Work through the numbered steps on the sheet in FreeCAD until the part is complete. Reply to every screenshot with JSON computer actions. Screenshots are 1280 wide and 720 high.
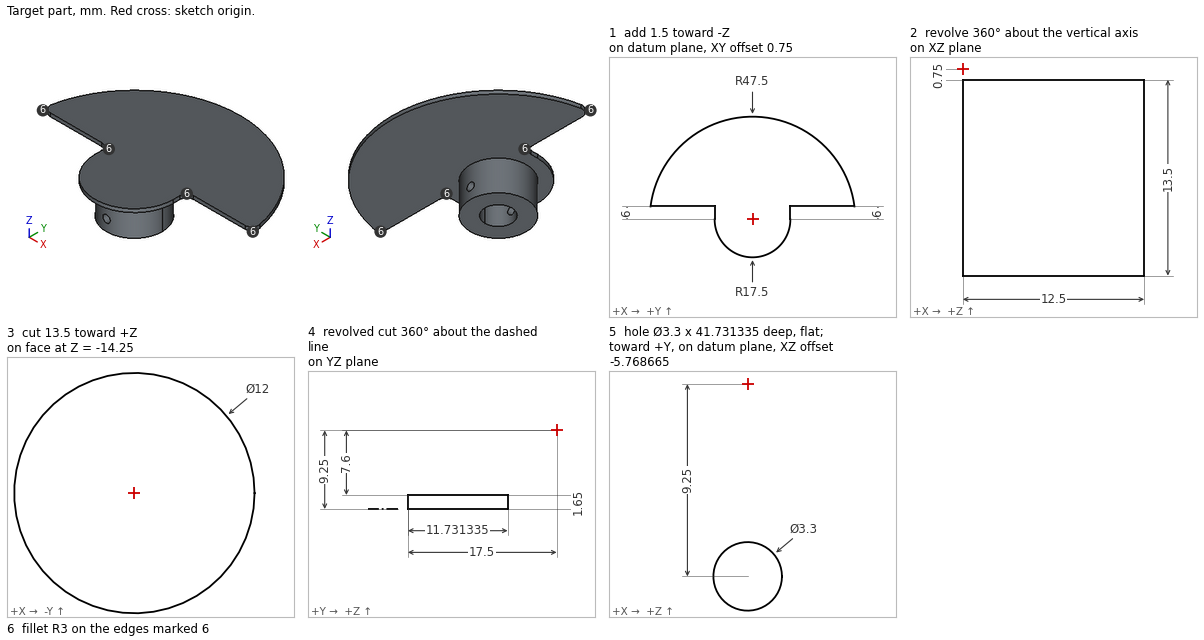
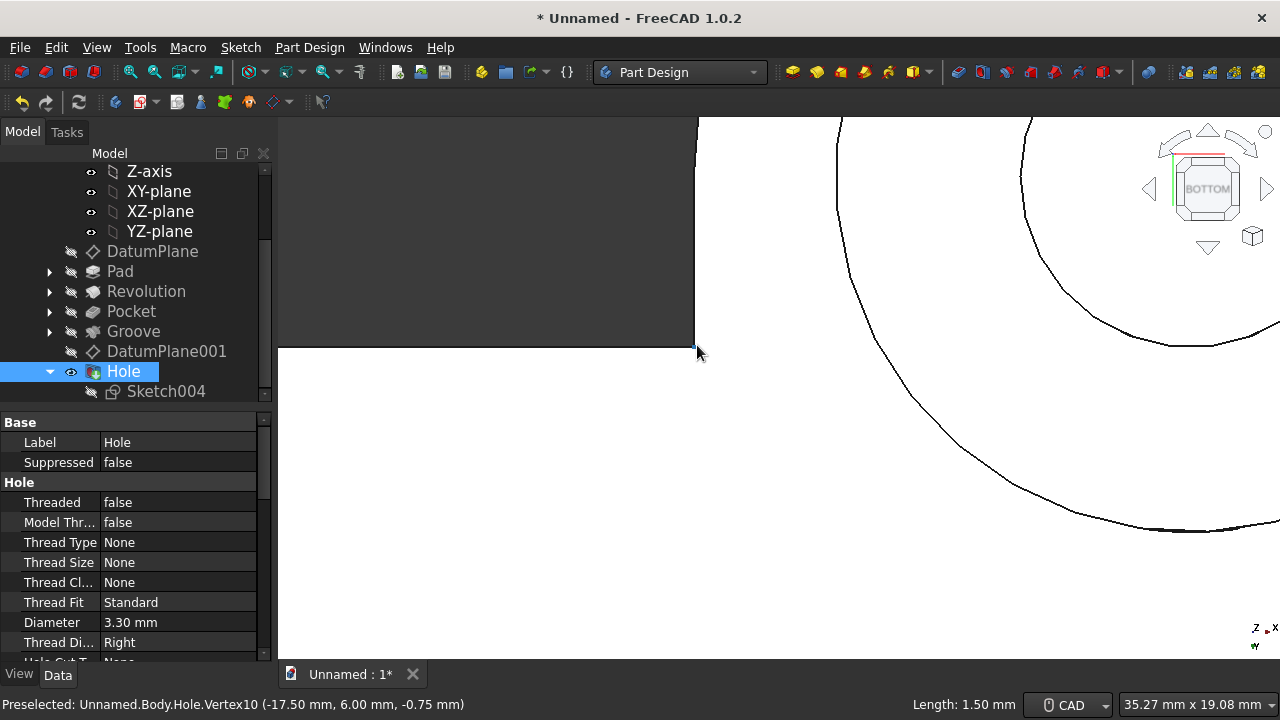
{"action": "key", "text": "v f"}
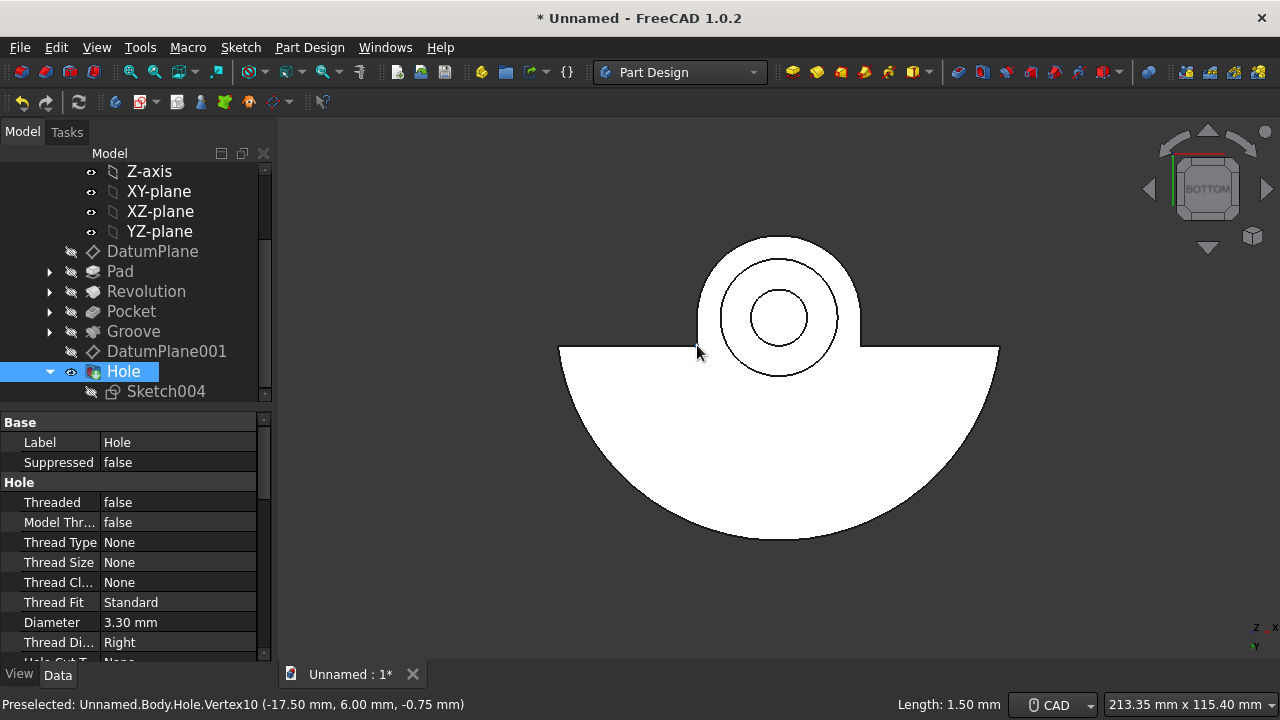
{"action": "key", "text": "4"}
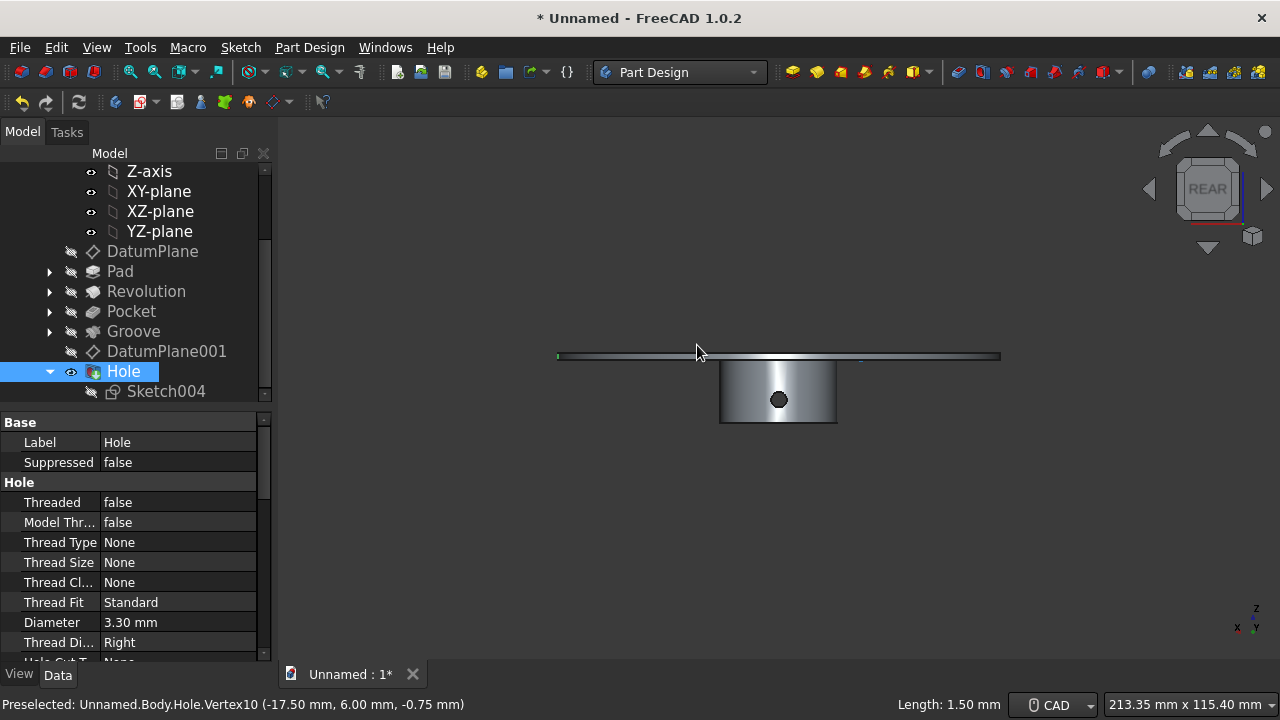
{"action": "left_click", "coordinate": [132, 72]}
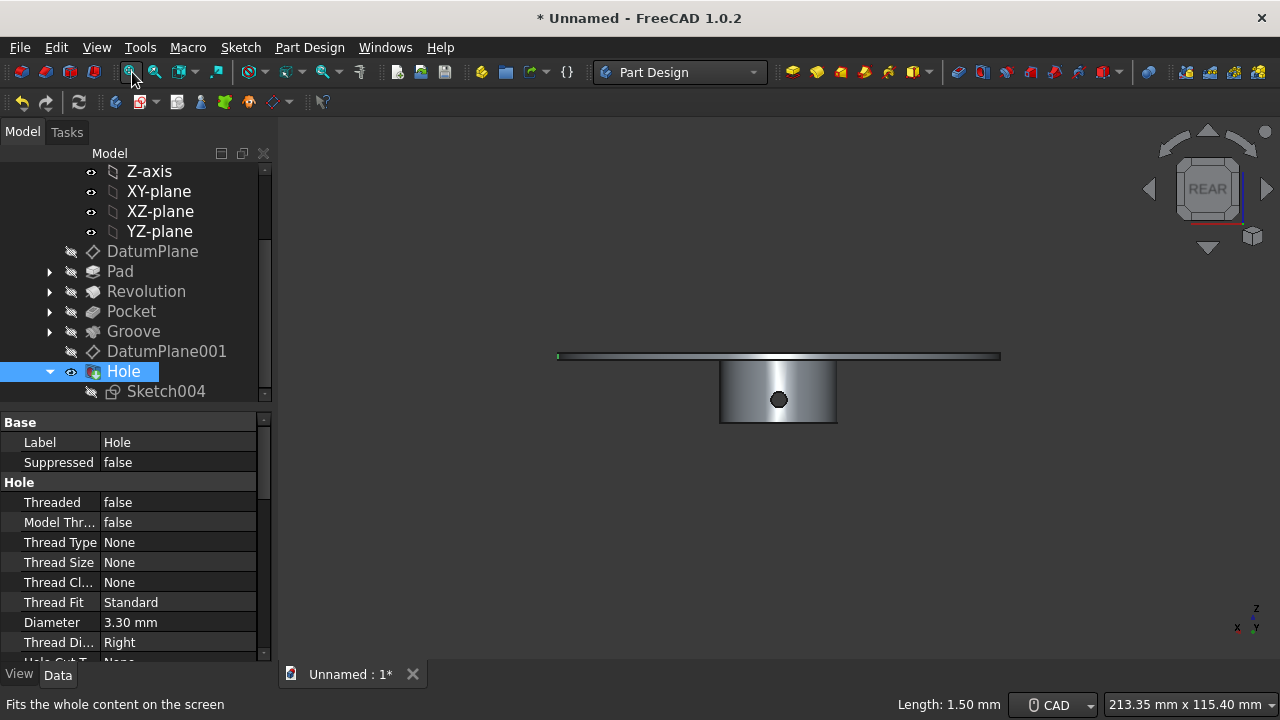
{"action": "scroll", "coordinate": [861, 355], "scroll_direction": "up", "scroll_amount": 9}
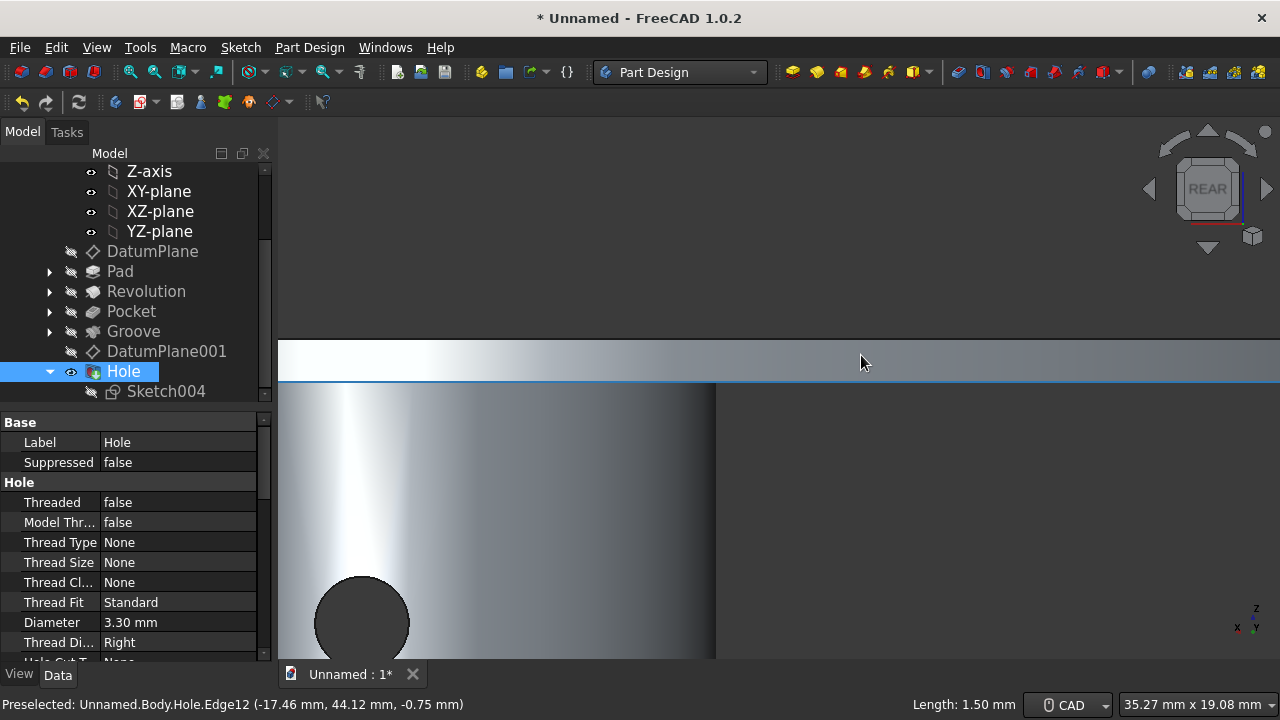
{"action": "key", "text": "v f"}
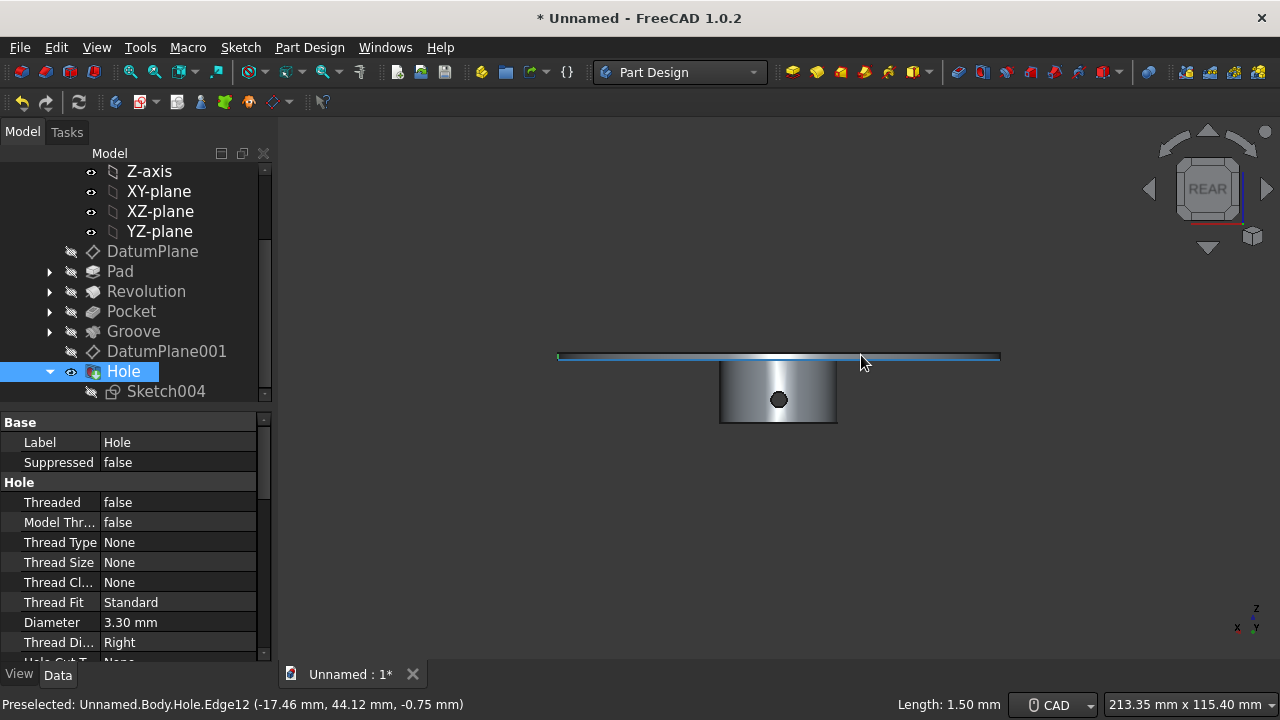
{"action": "key", "text": "6"}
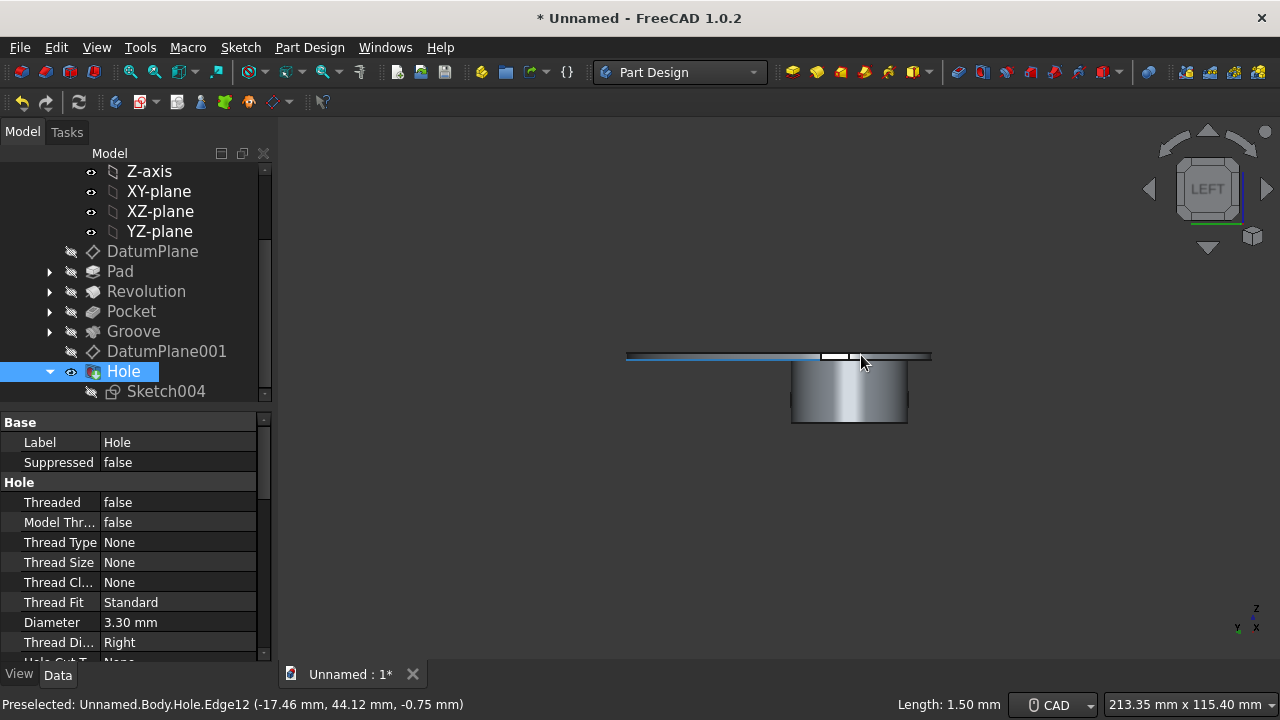
{"action": "key", "text": "v f"}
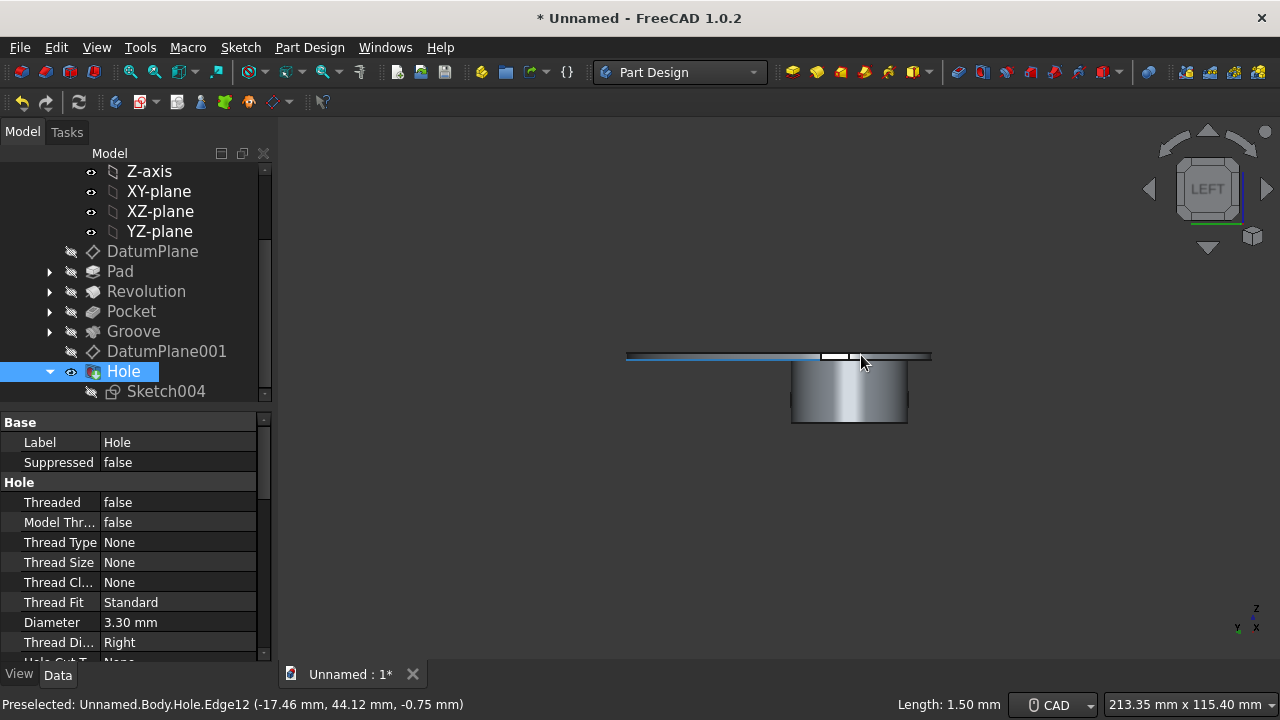
{"action": "scroll", "coordinate": [821, 355], "scroll_direction": "up", "scroll_amount": 9}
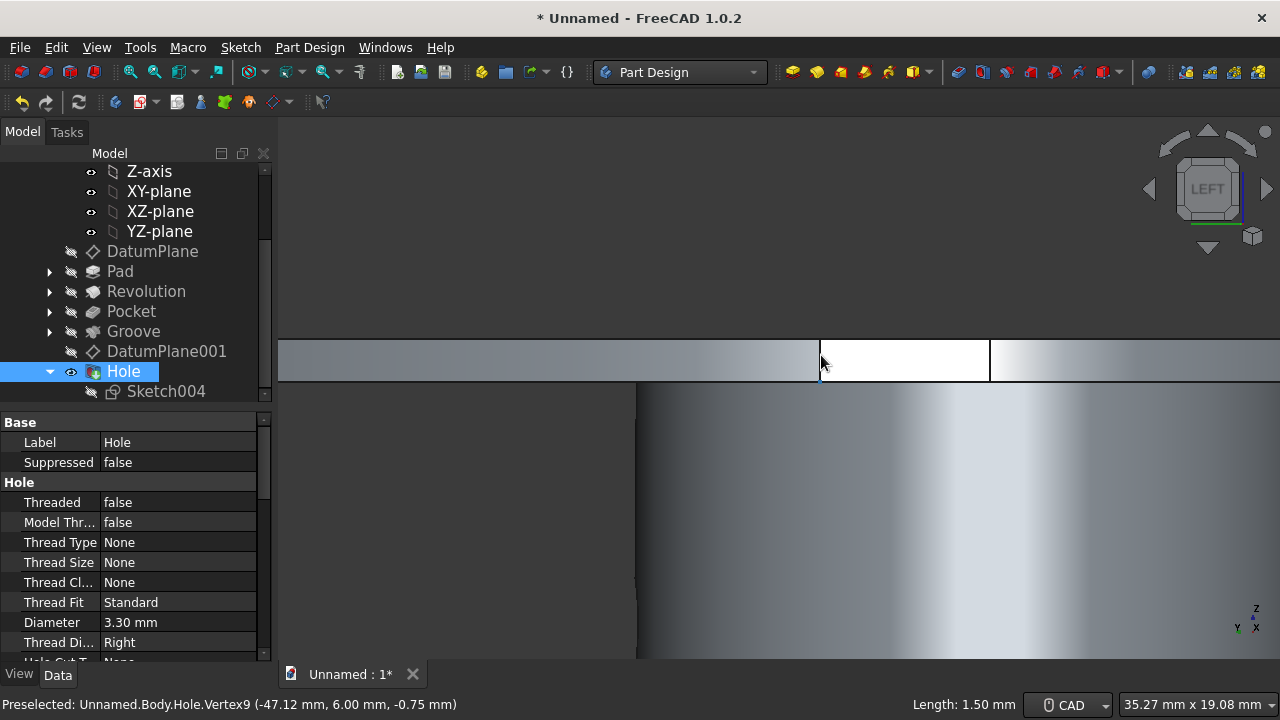
{"action": "left_click", "coordinate": [820, 360], "text": "ctrl"}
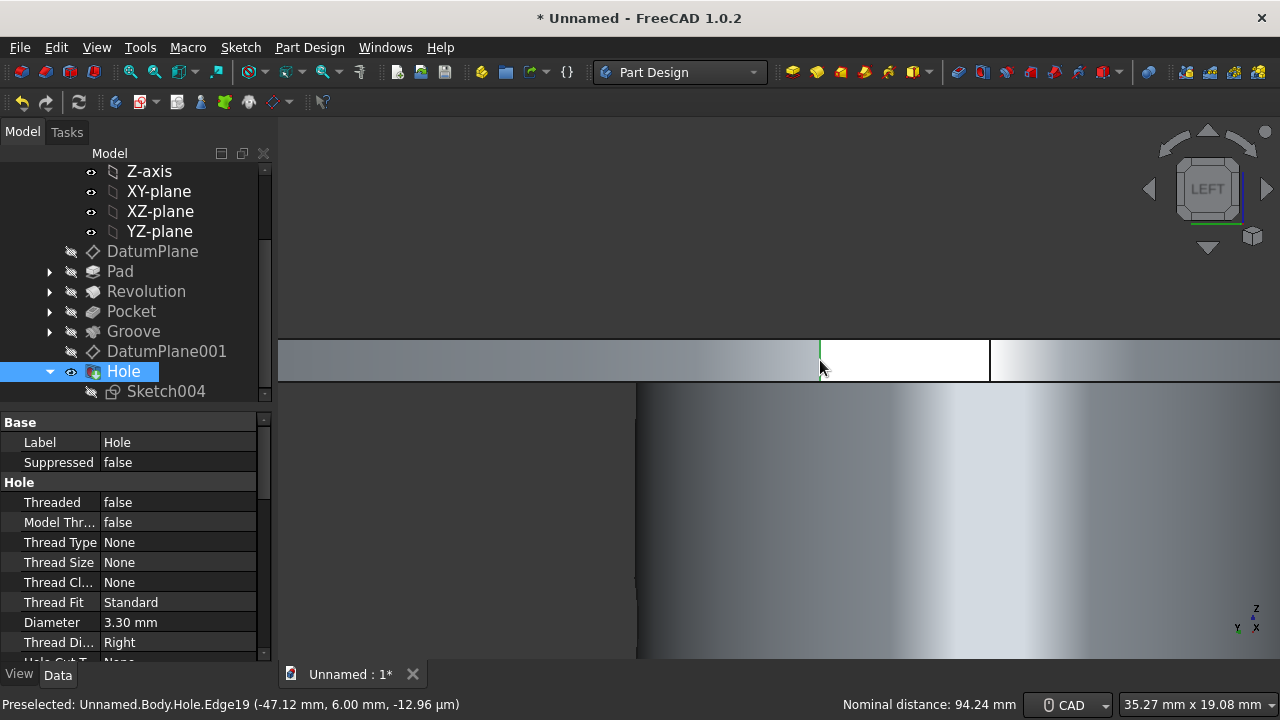
{"action": "key", "text": "v f"}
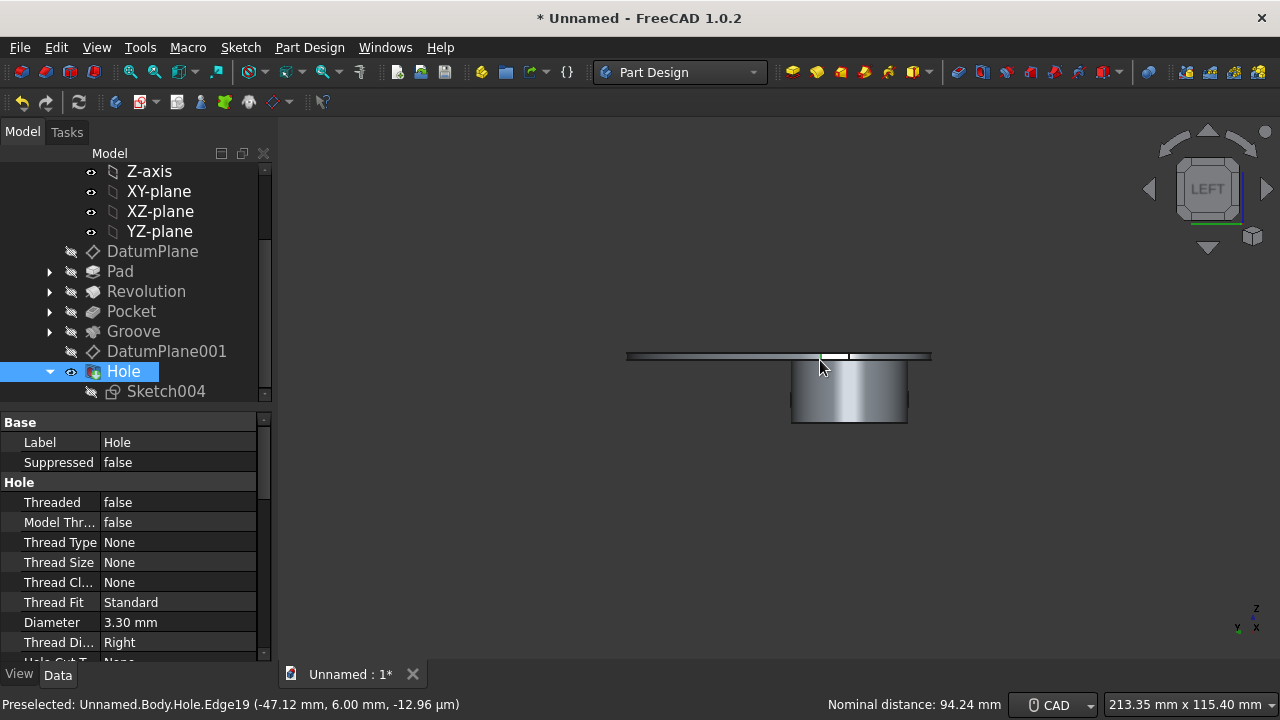
{"action": "key", "text": "v 3"}